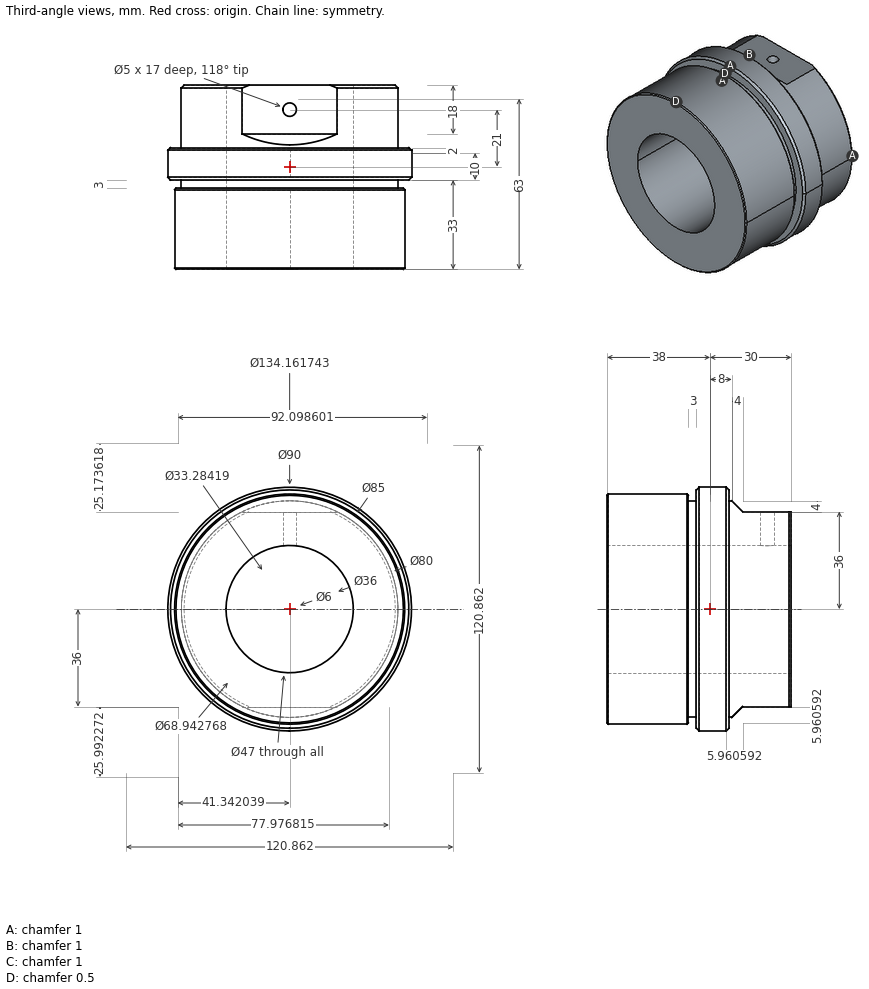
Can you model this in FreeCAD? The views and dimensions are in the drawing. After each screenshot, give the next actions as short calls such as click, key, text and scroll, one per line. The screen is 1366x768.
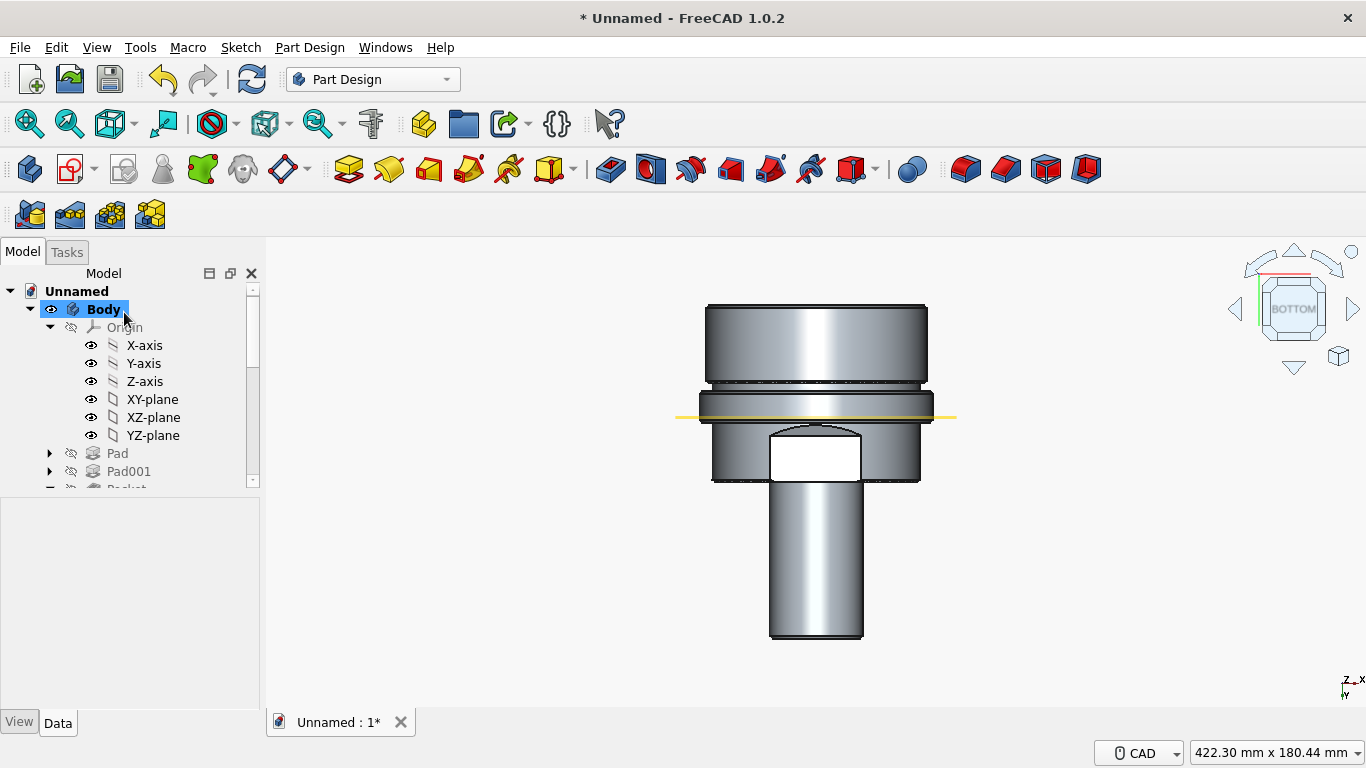
scroll(100, 377, down, 3)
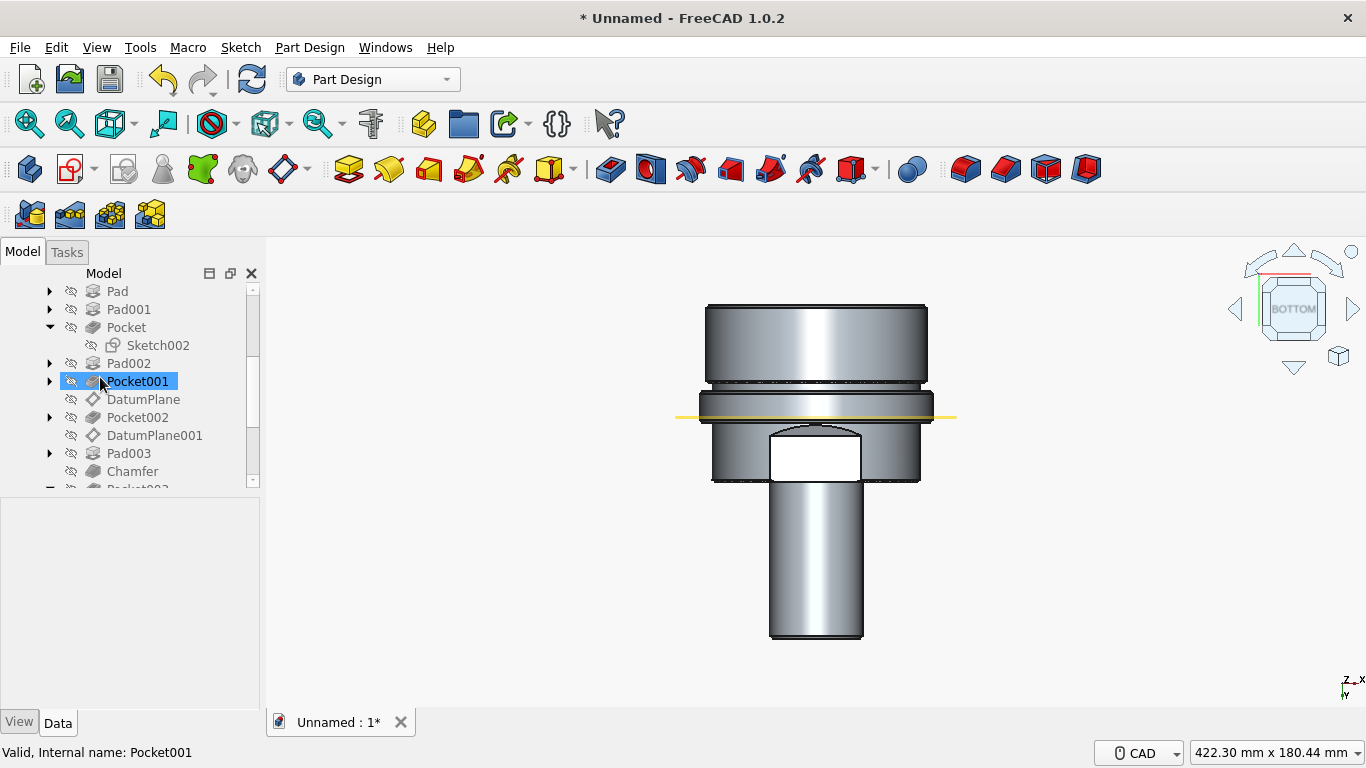
scroll(140, 377, up, 15)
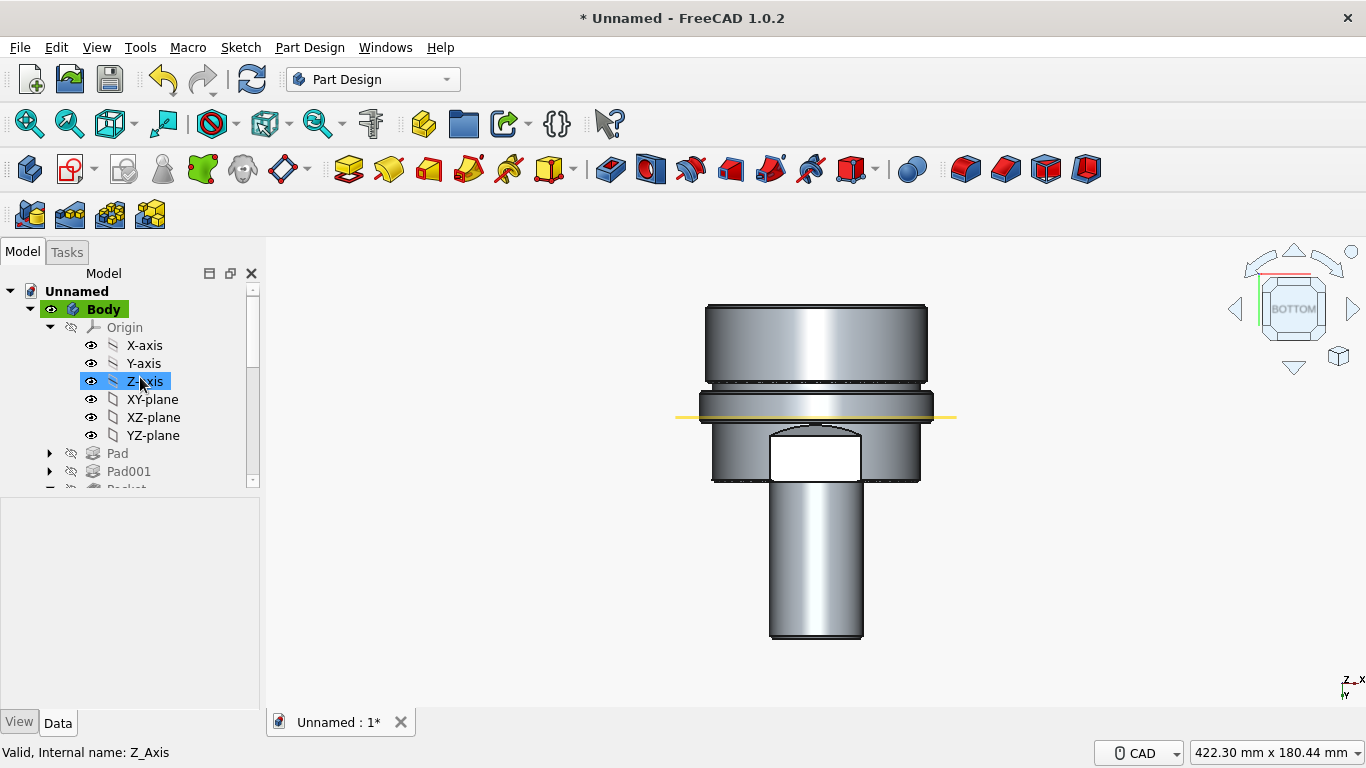
scroll(100, 377, down, 6)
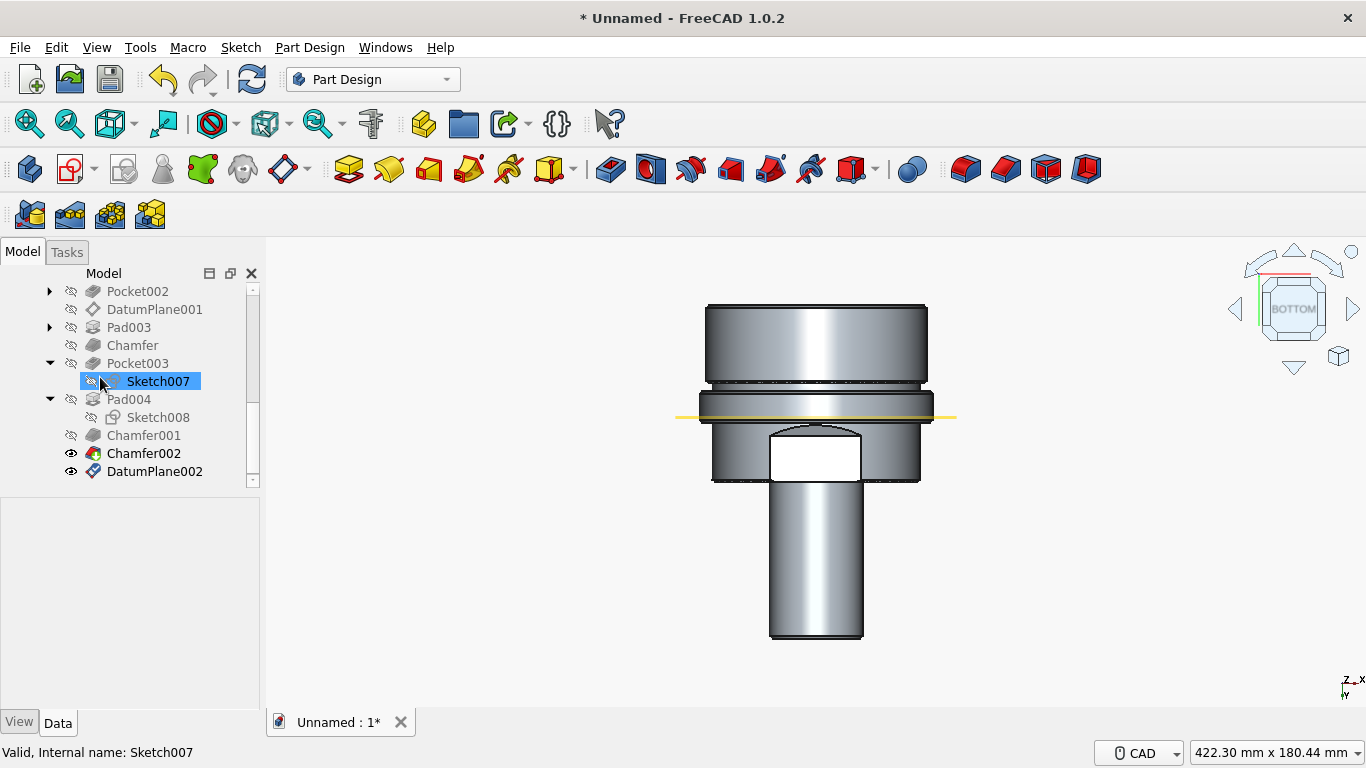
click(116, 471)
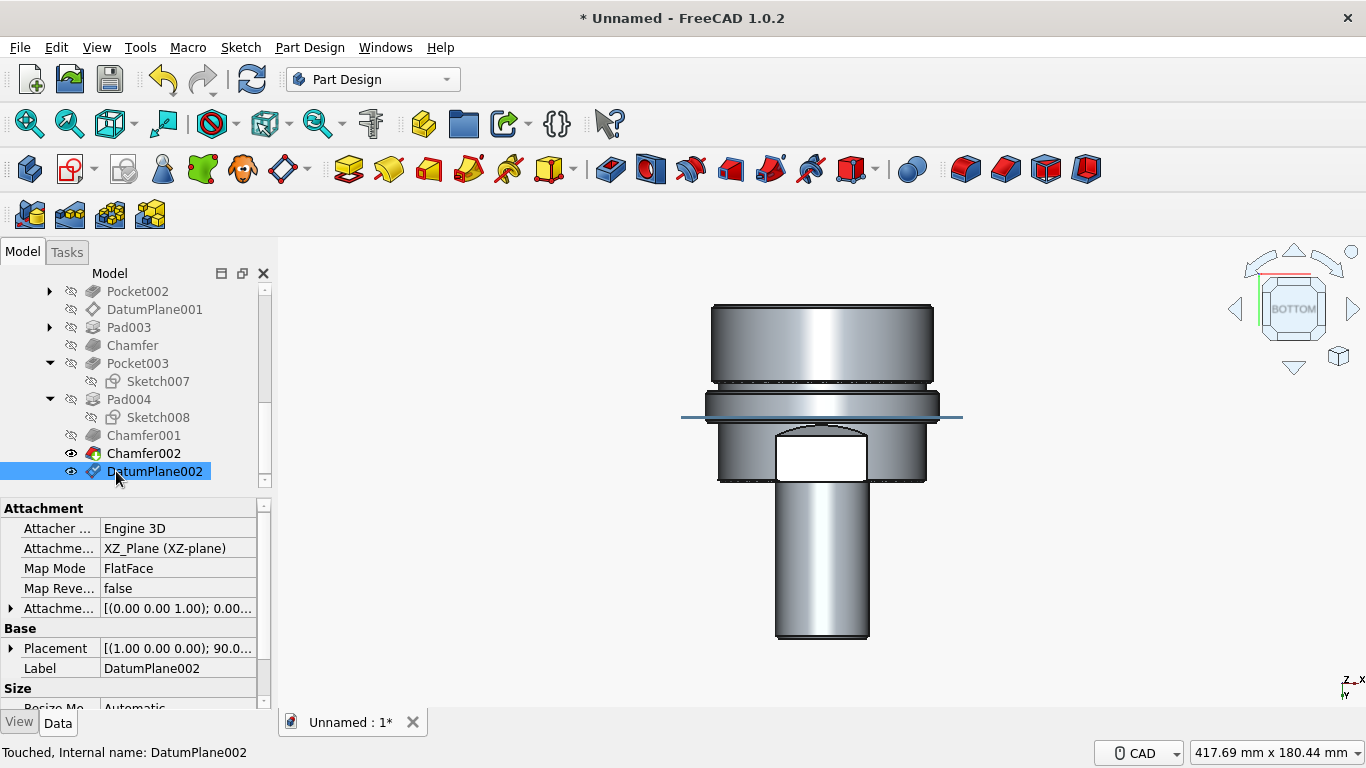
click(70, 170)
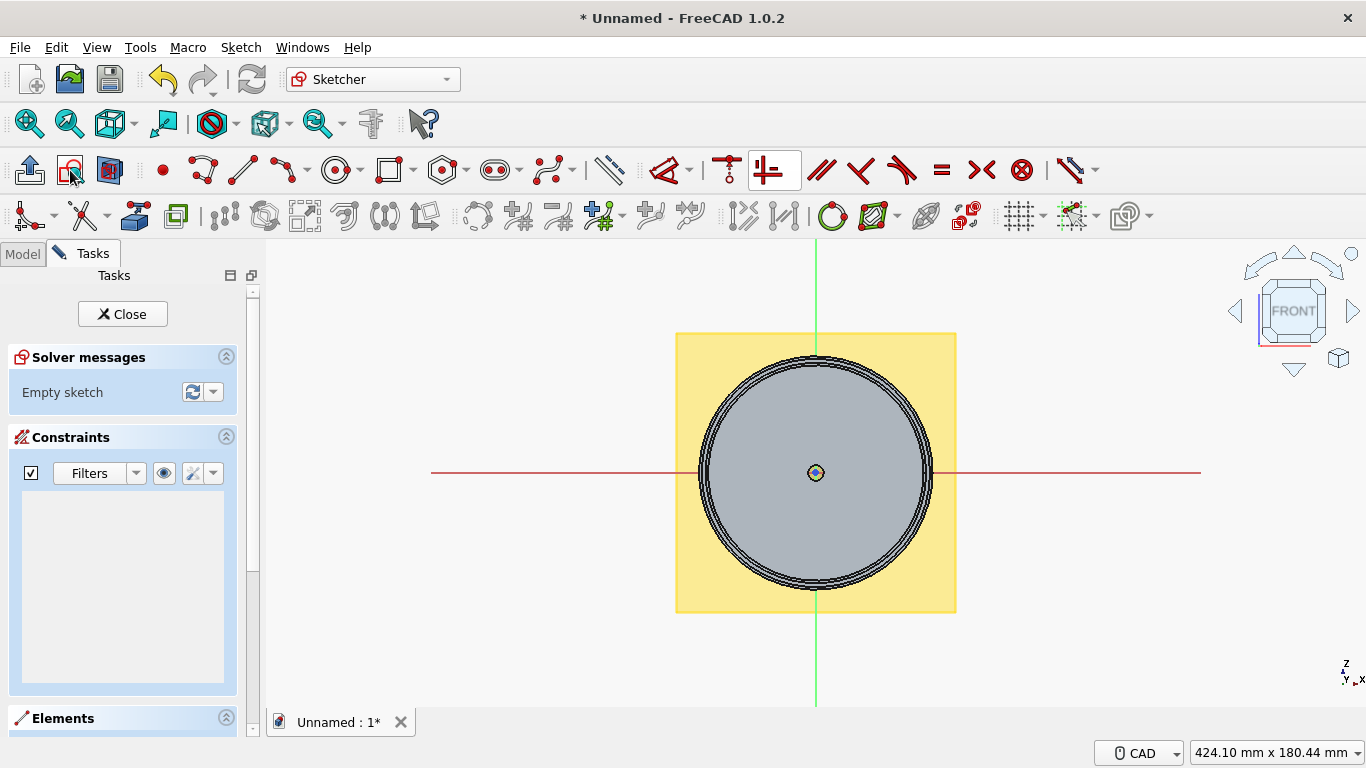
click(110, 170)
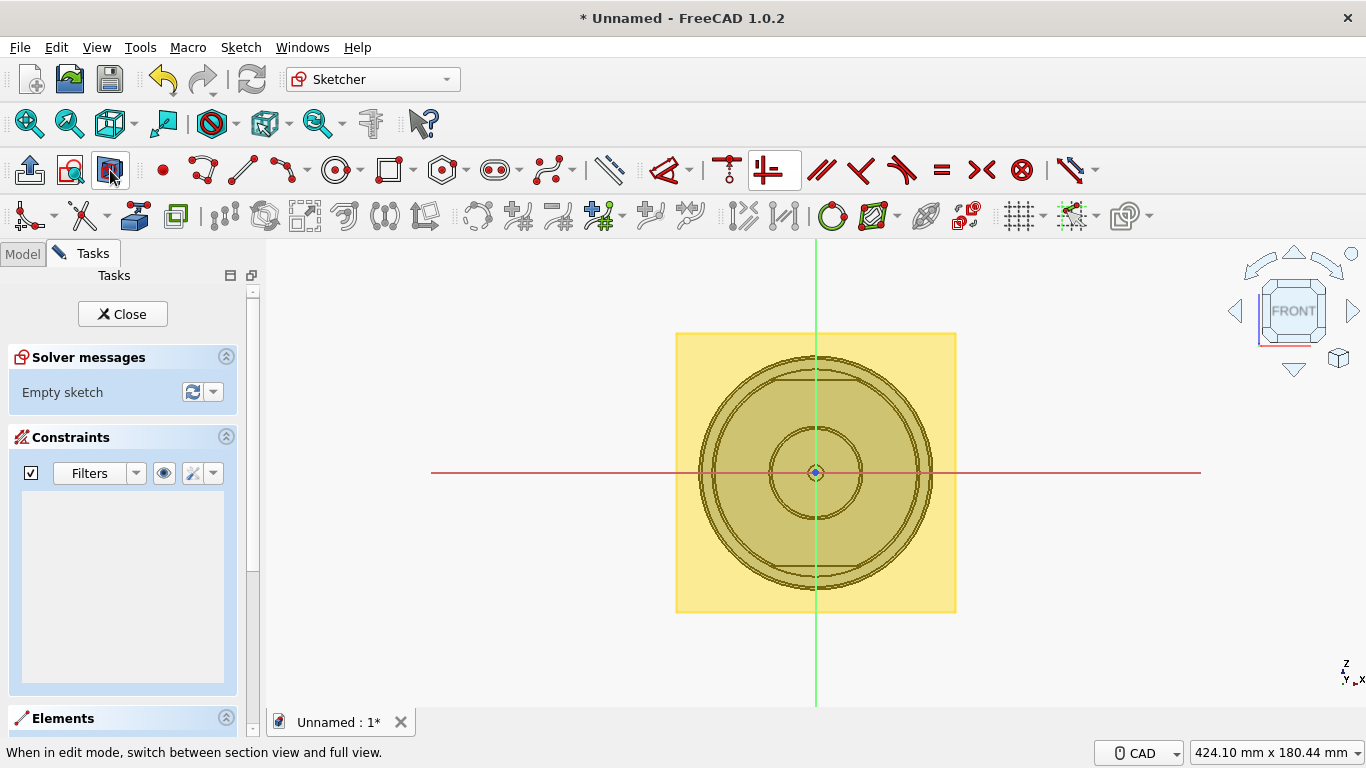
scroll(819, 473, up, 15)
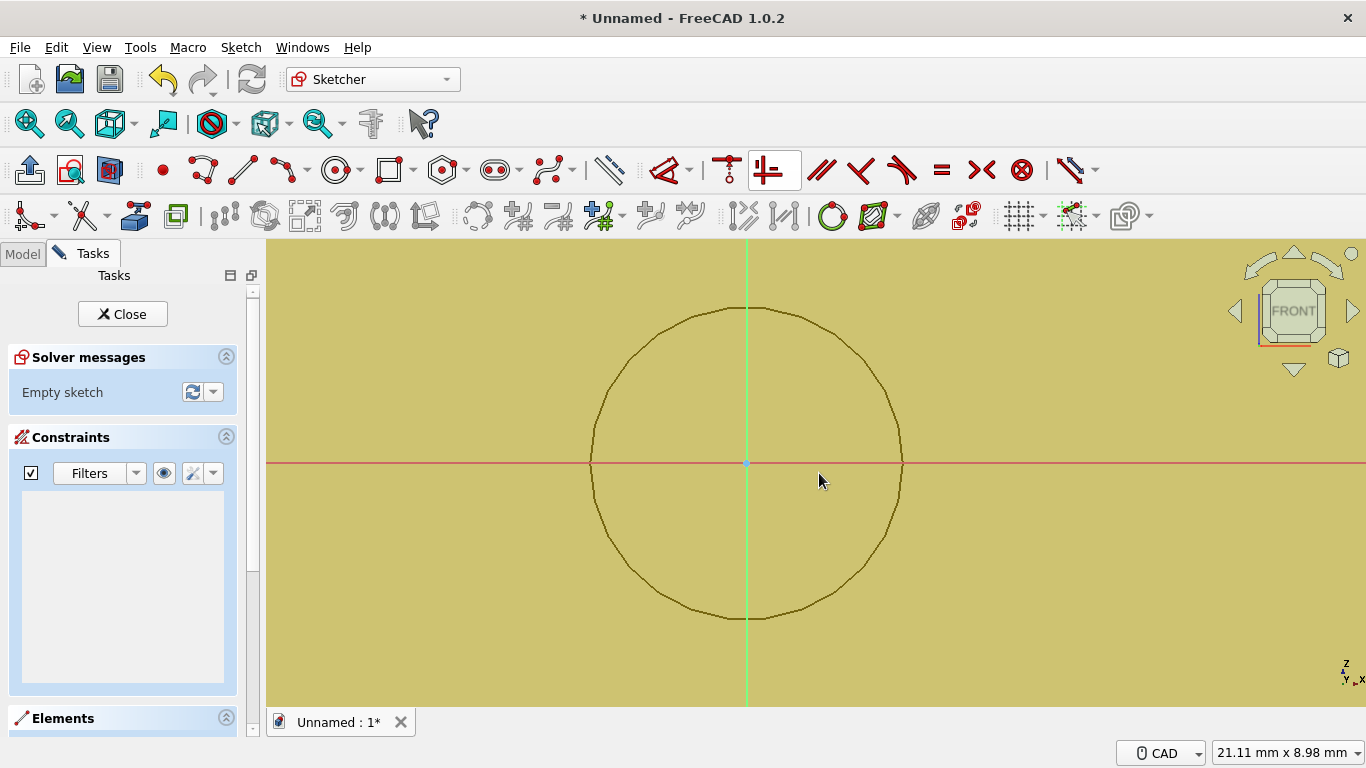
click(336, 170)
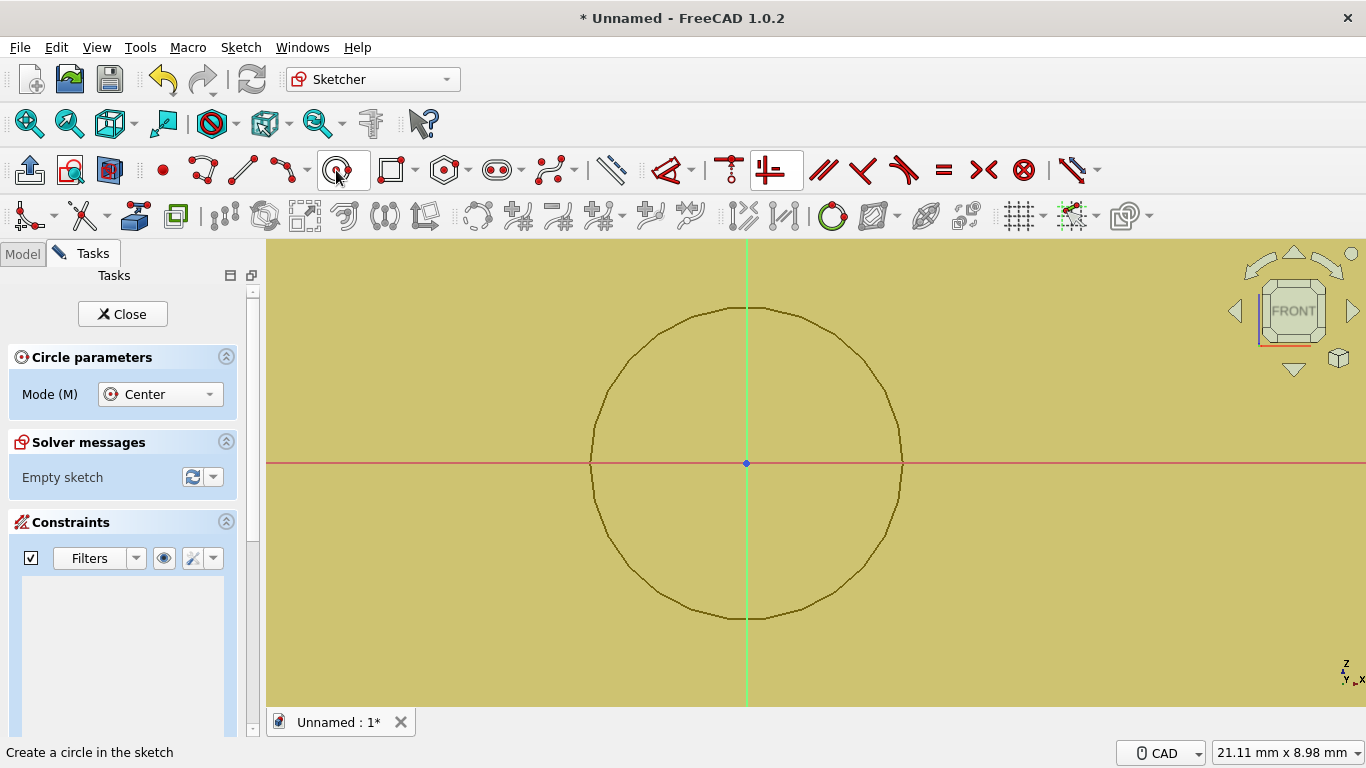
click(747, 463)
click(857, 353)
key(Escape)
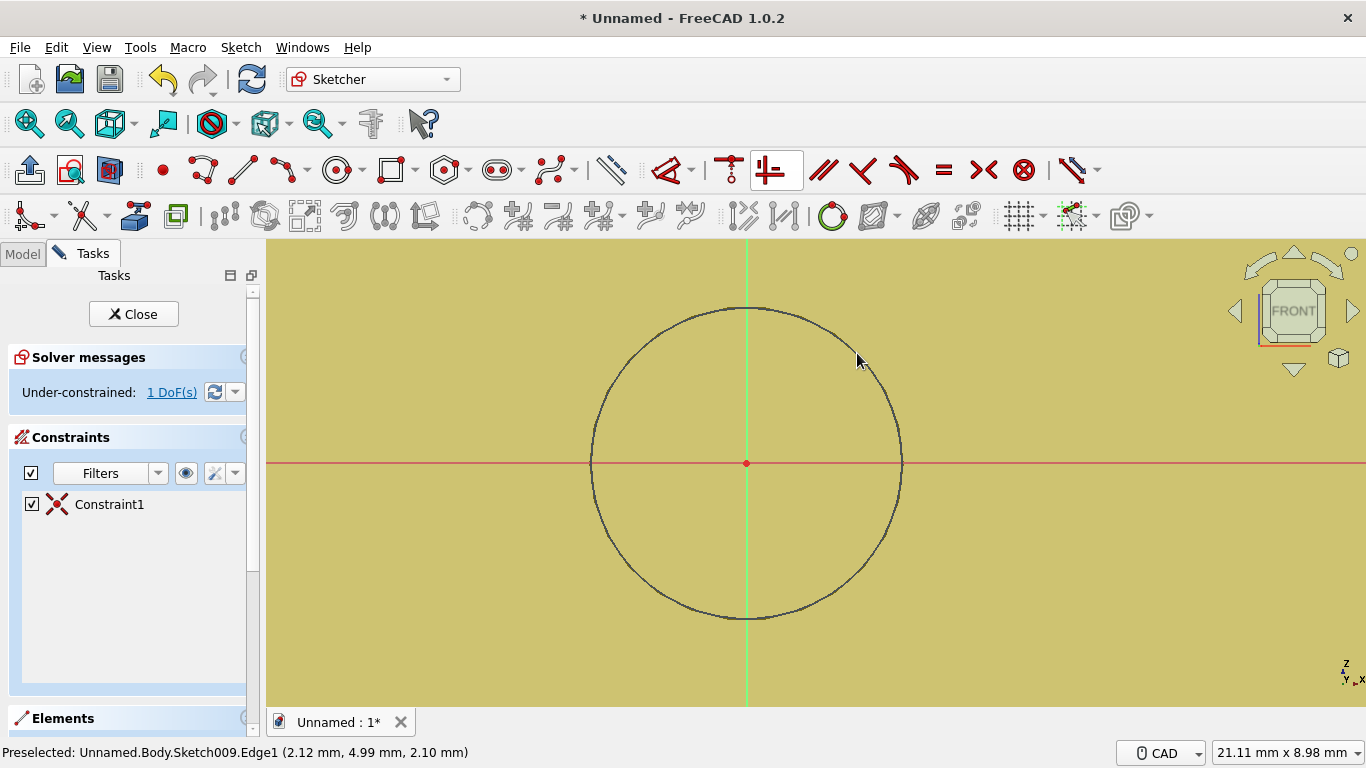
click(666, 170)